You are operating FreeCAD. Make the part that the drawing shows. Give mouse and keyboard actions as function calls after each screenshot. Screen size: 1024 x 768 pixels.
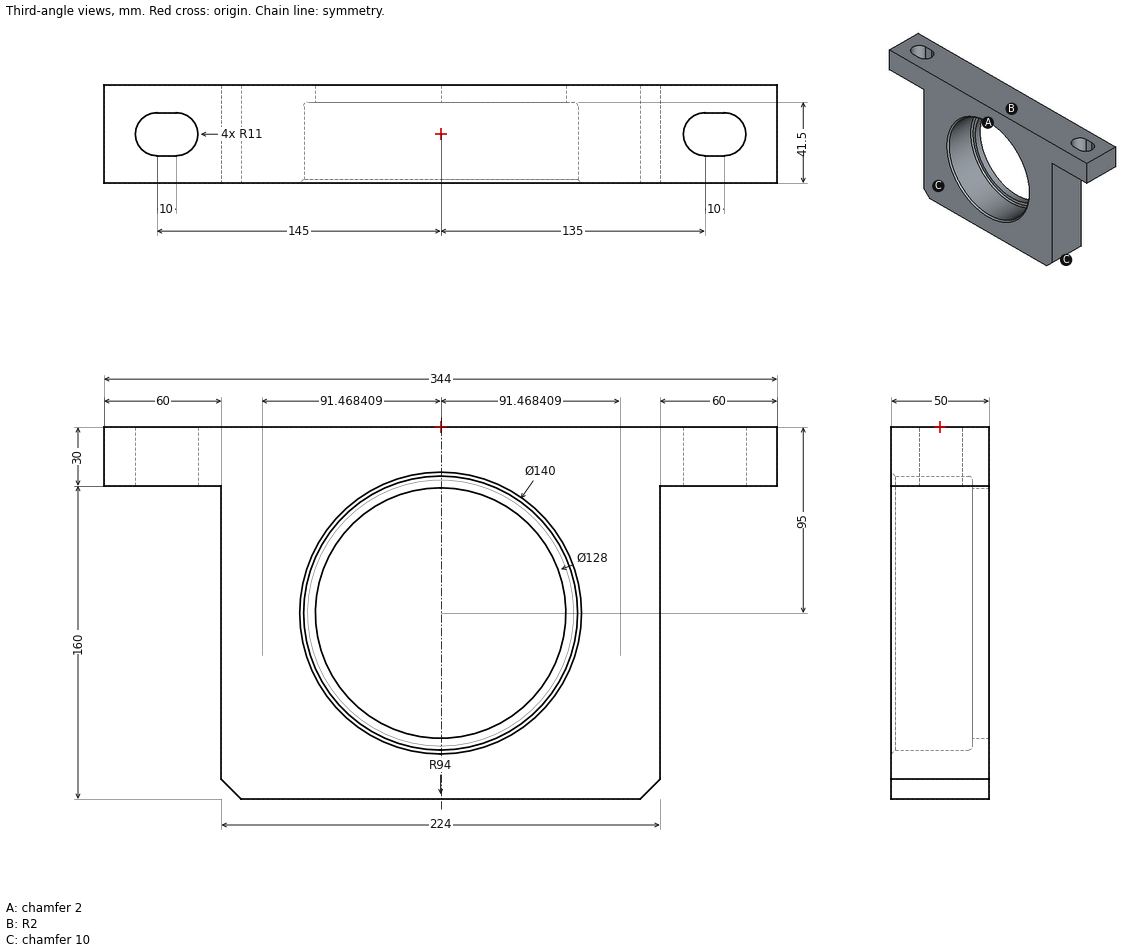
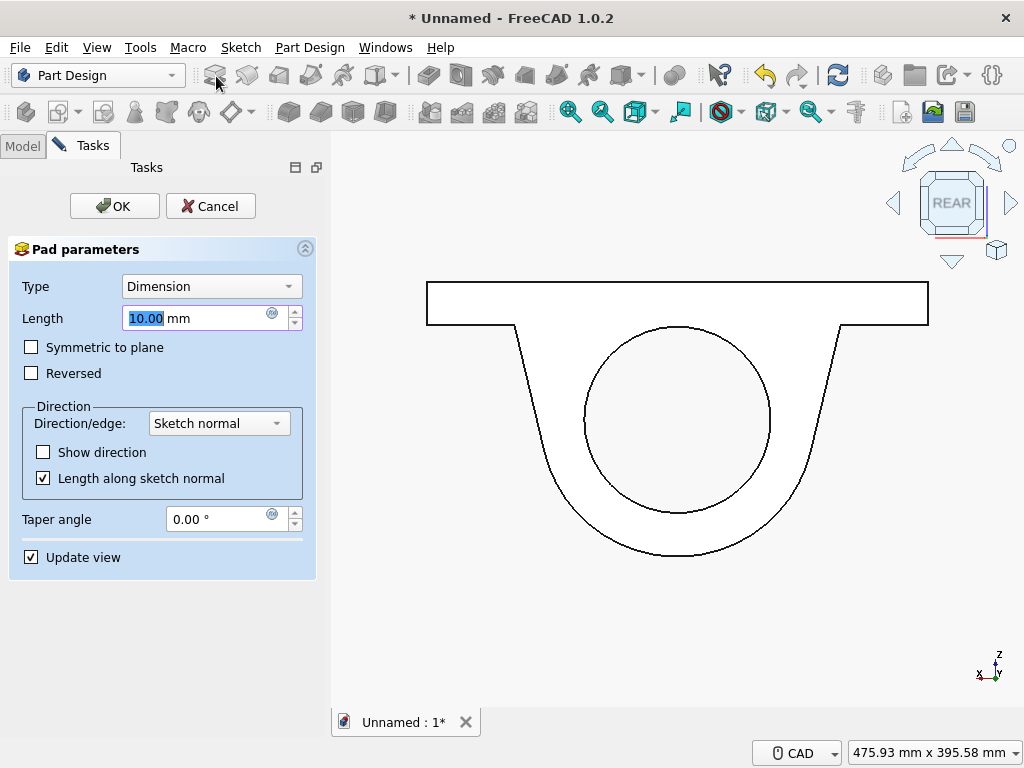
text(50)
key(Tab)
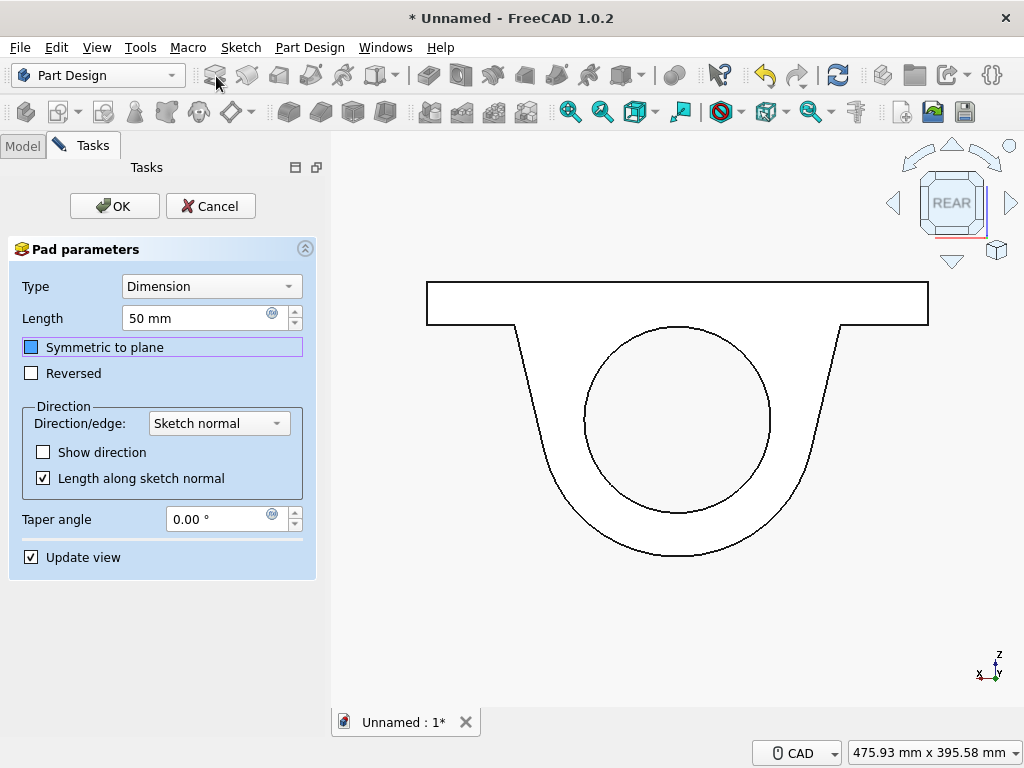
click(30, 373)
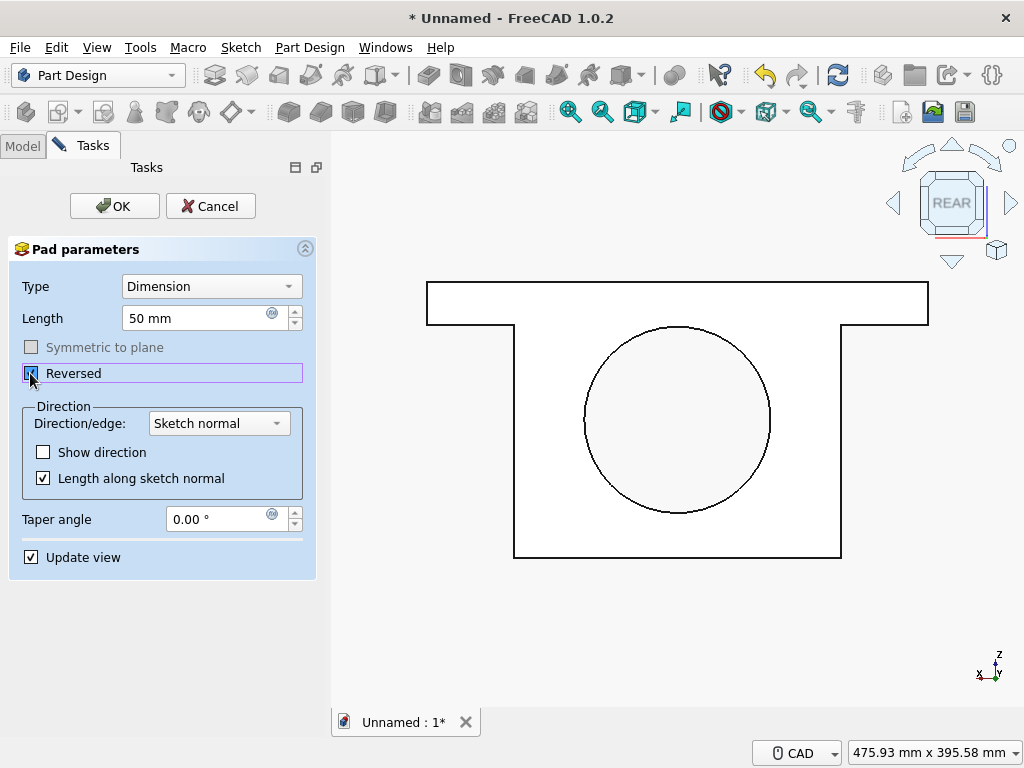
click(115, 206)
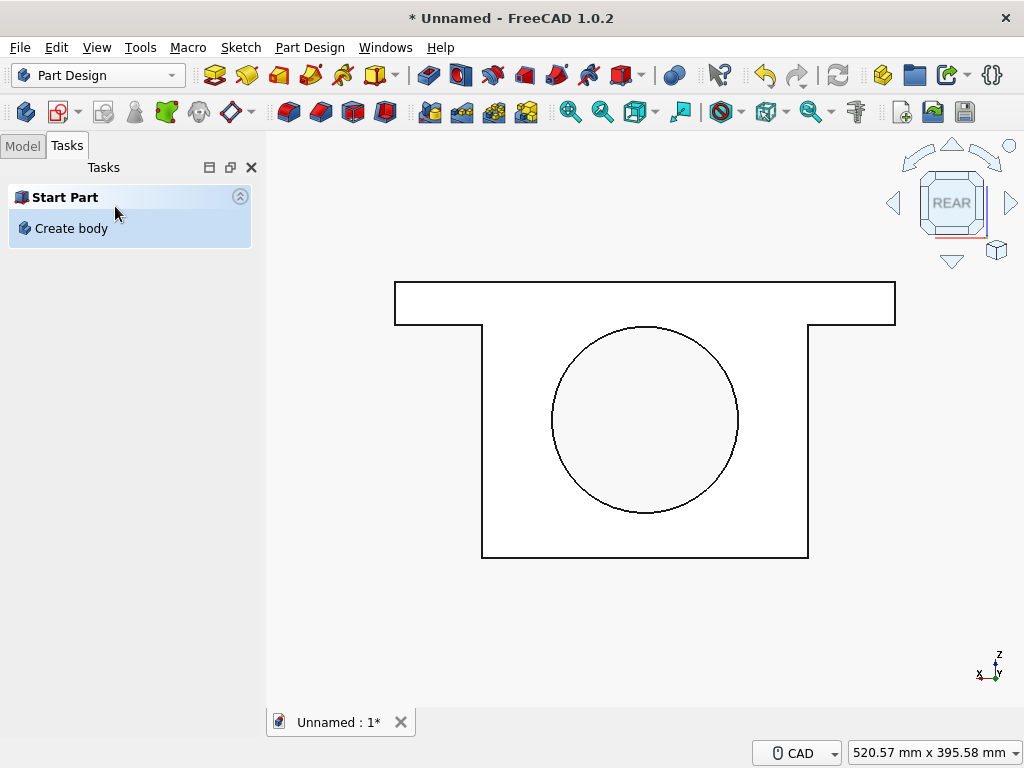
key(0)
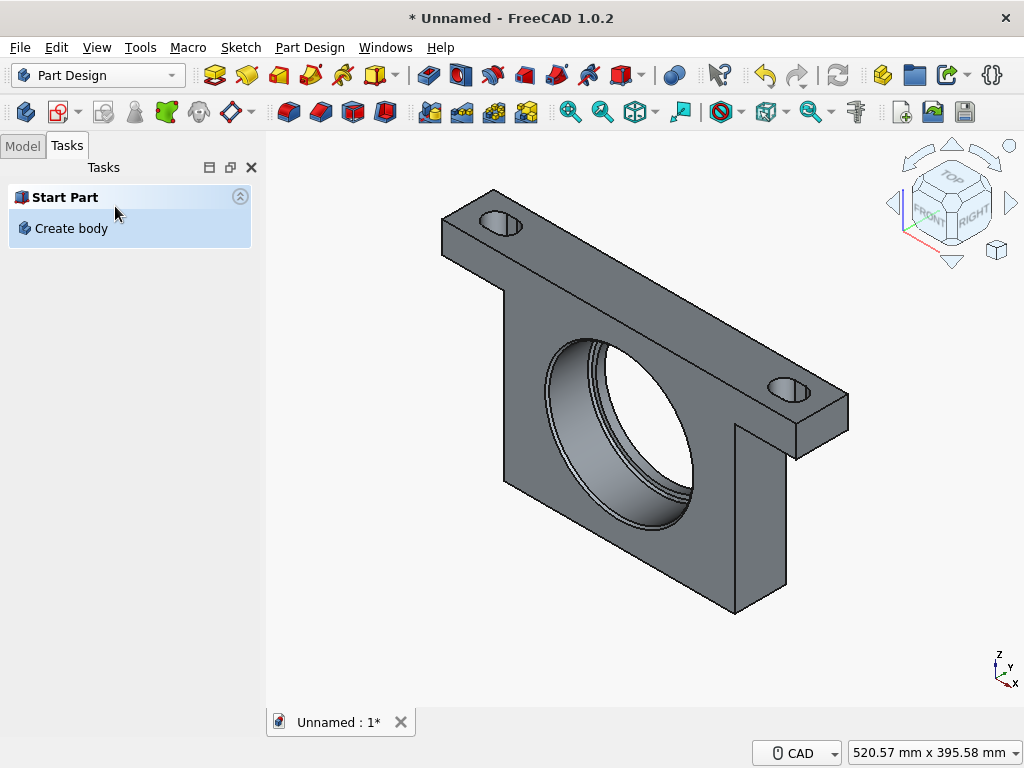
key(2)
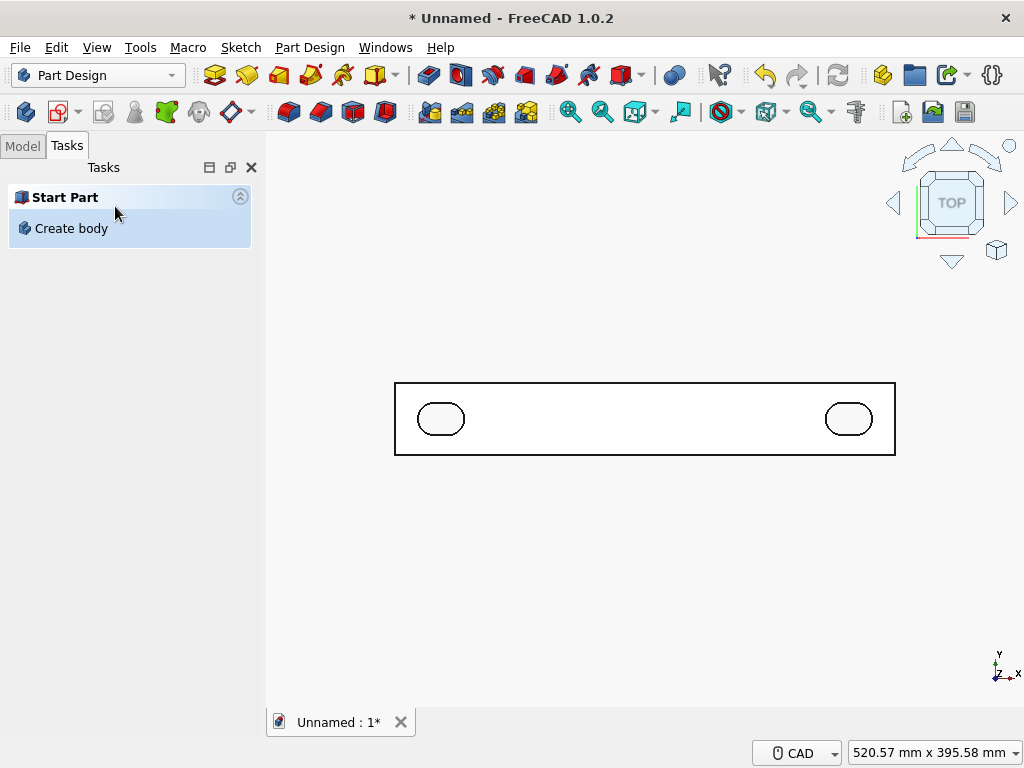
key(1)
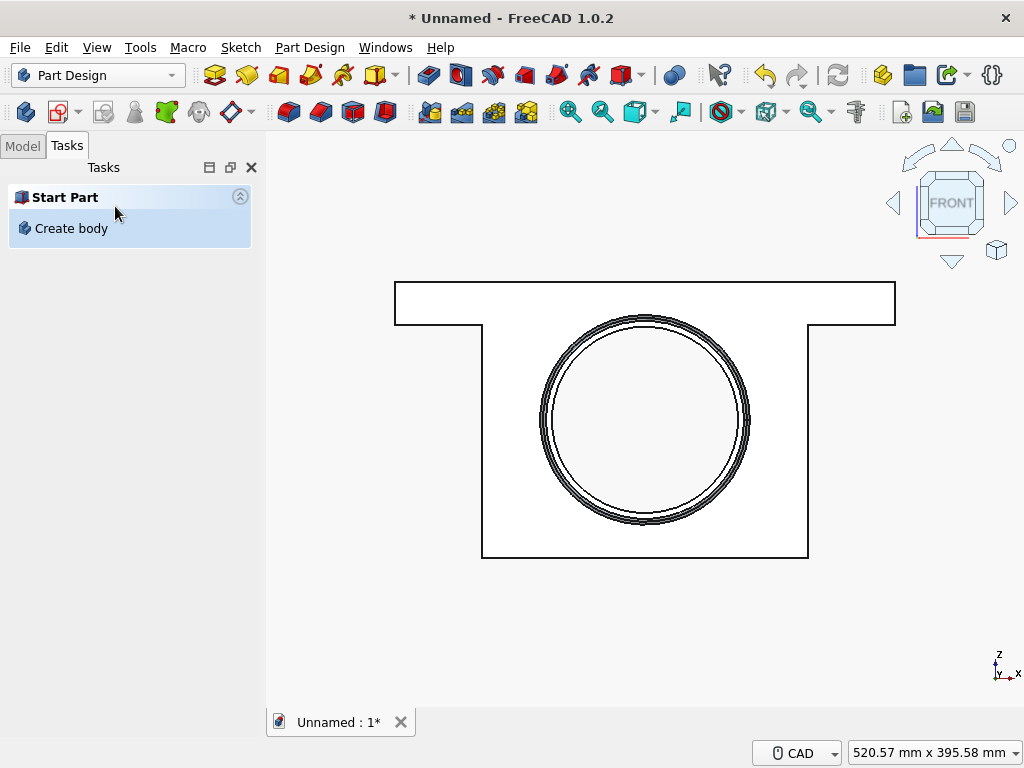
key(3)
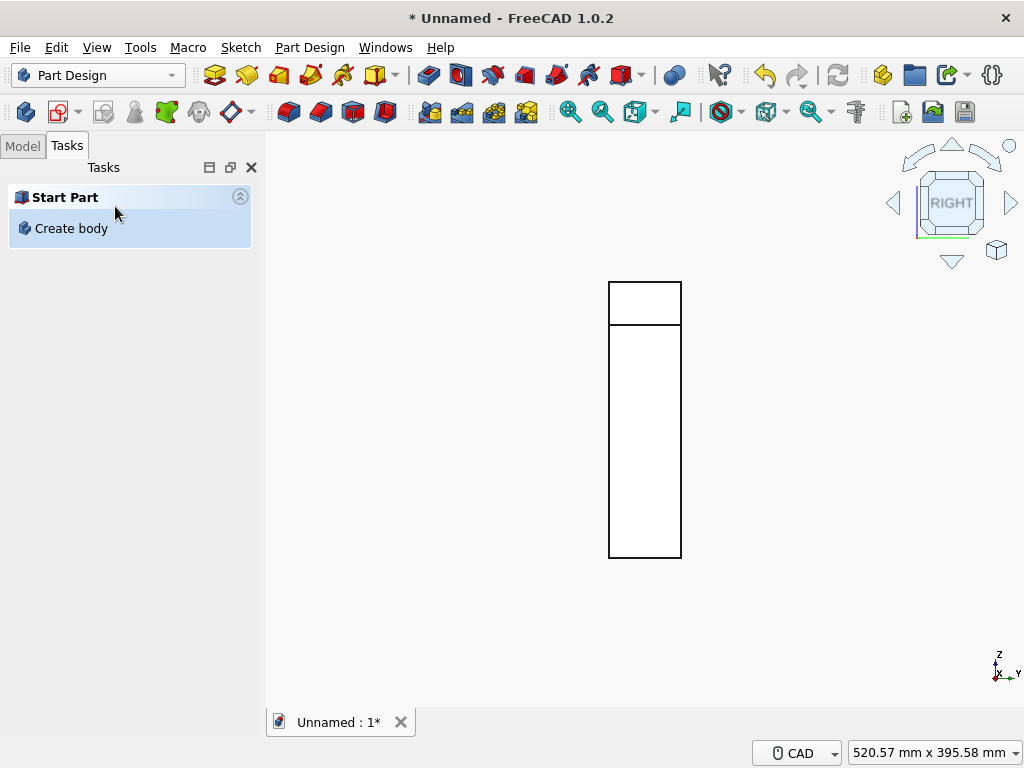
click(645, 557)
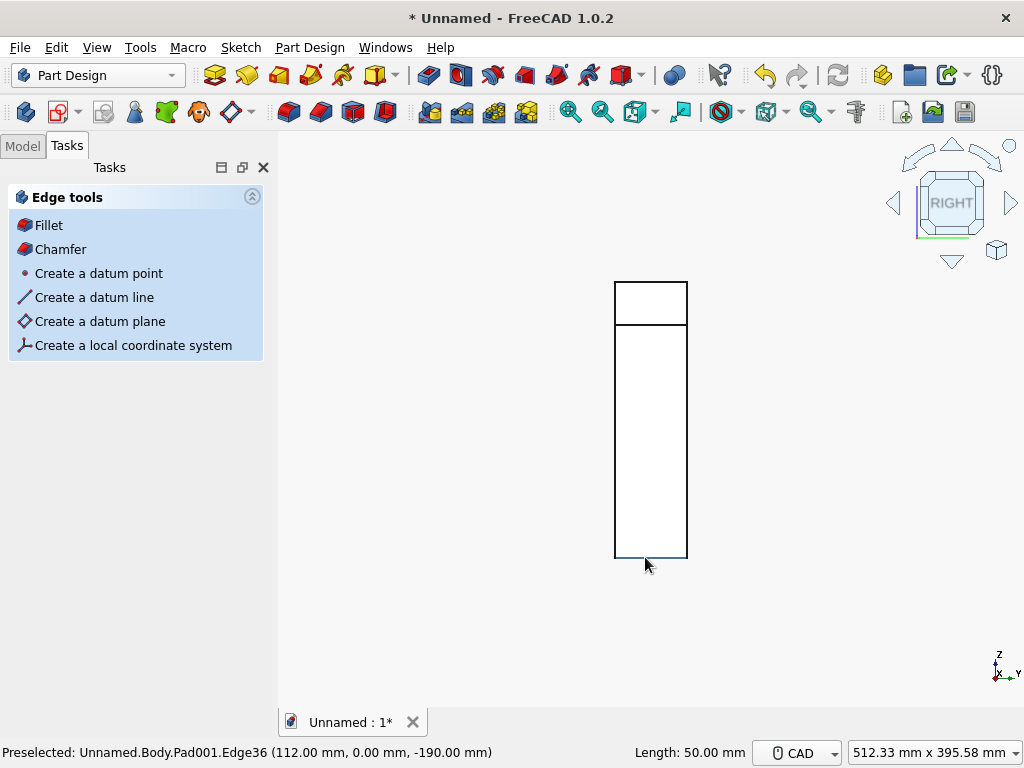
key(5)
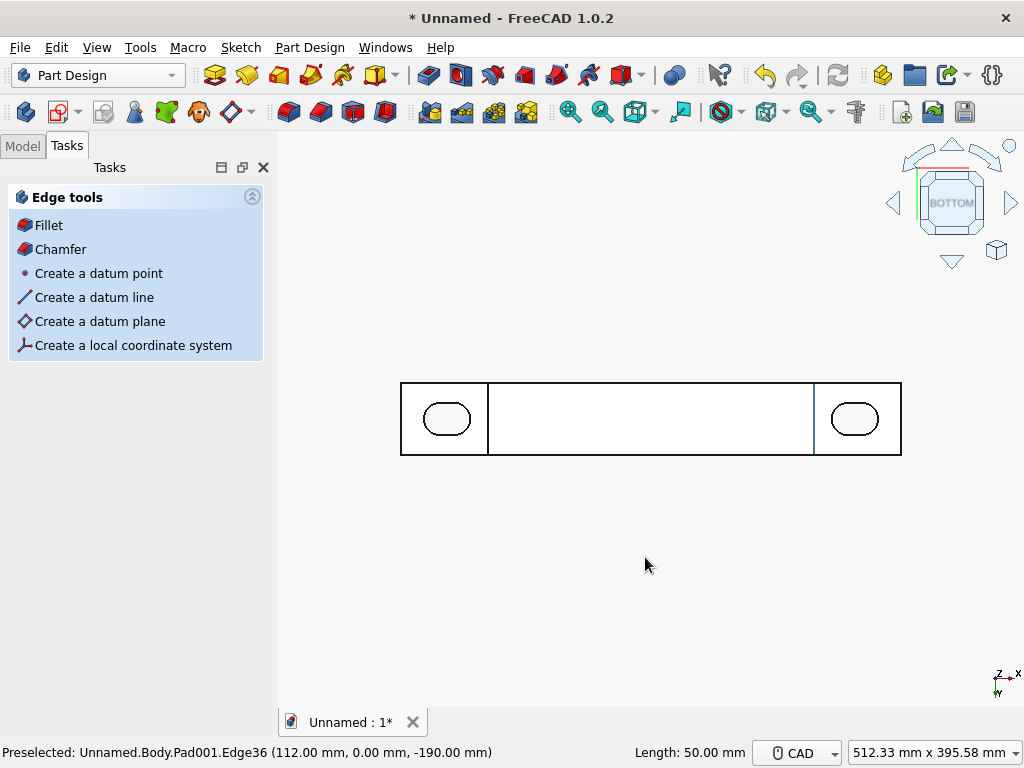
click(488, 418, ctrl)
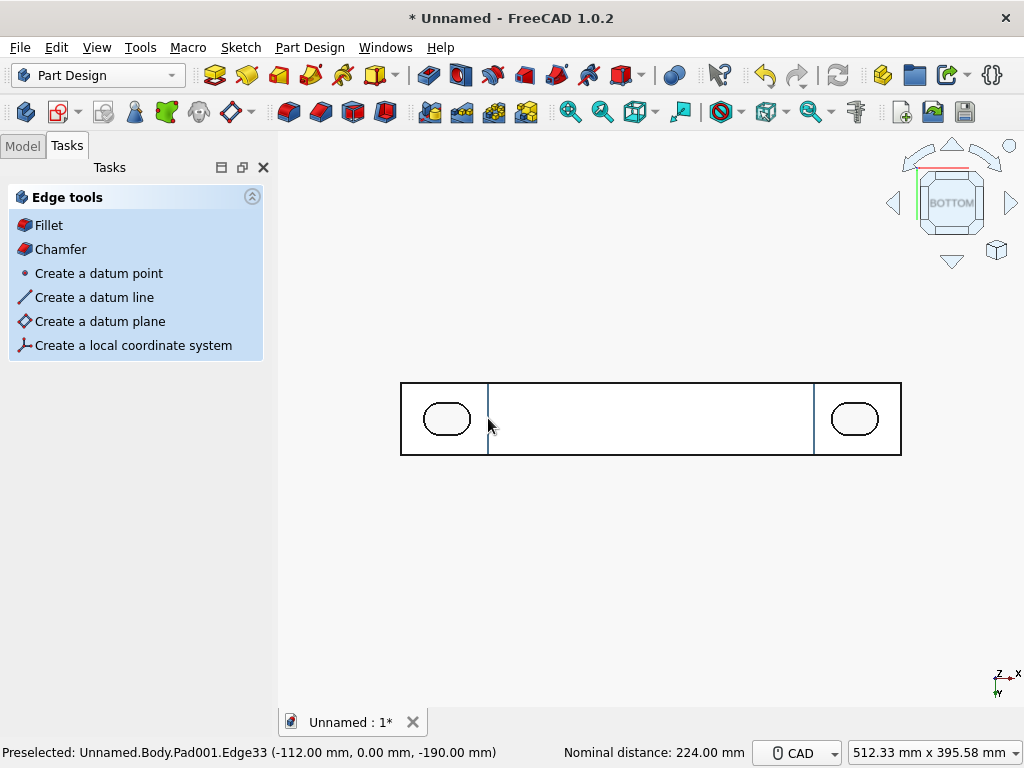
click(322, 112)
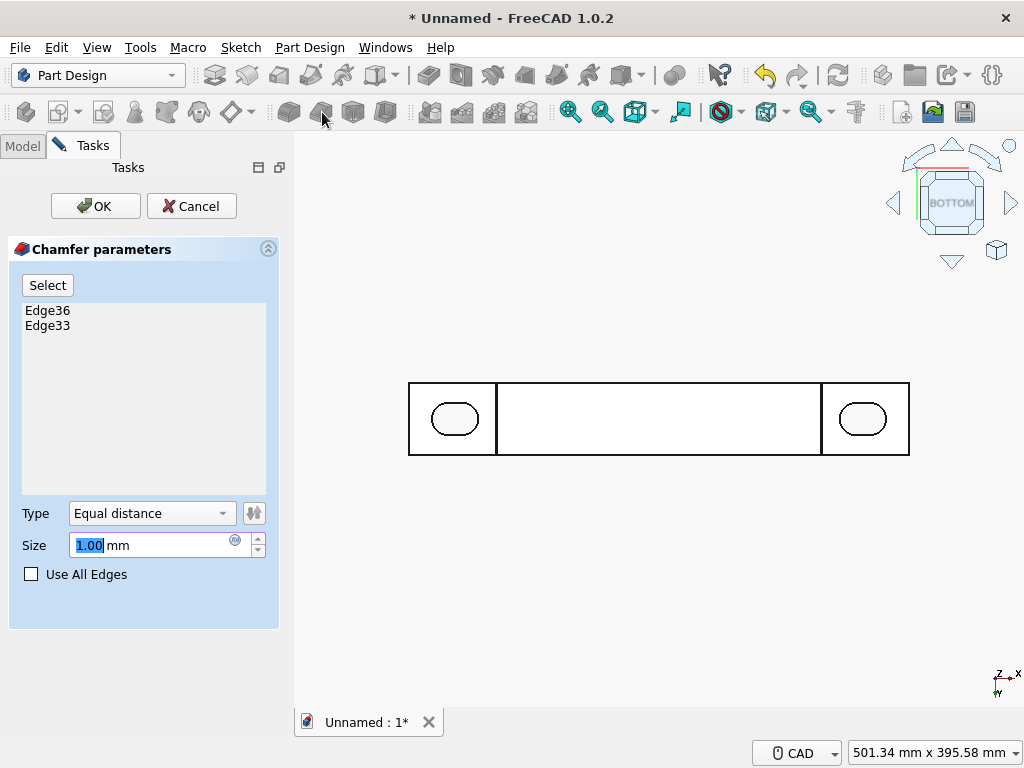
text(10)
key(Tab)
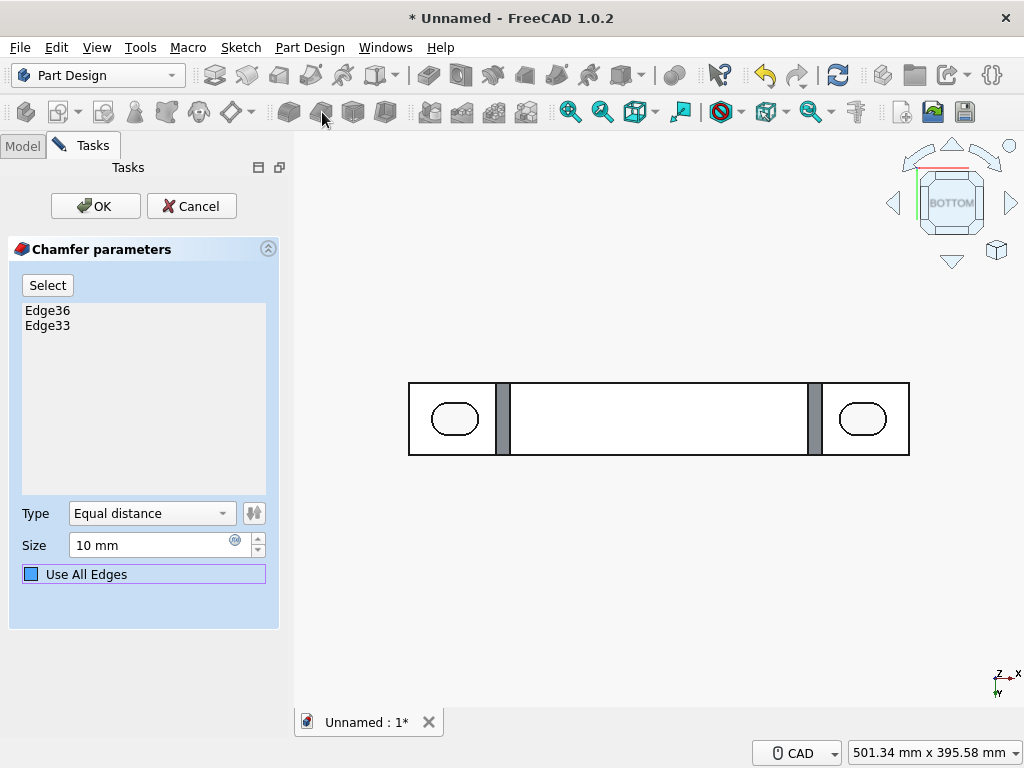
click(96, 206)